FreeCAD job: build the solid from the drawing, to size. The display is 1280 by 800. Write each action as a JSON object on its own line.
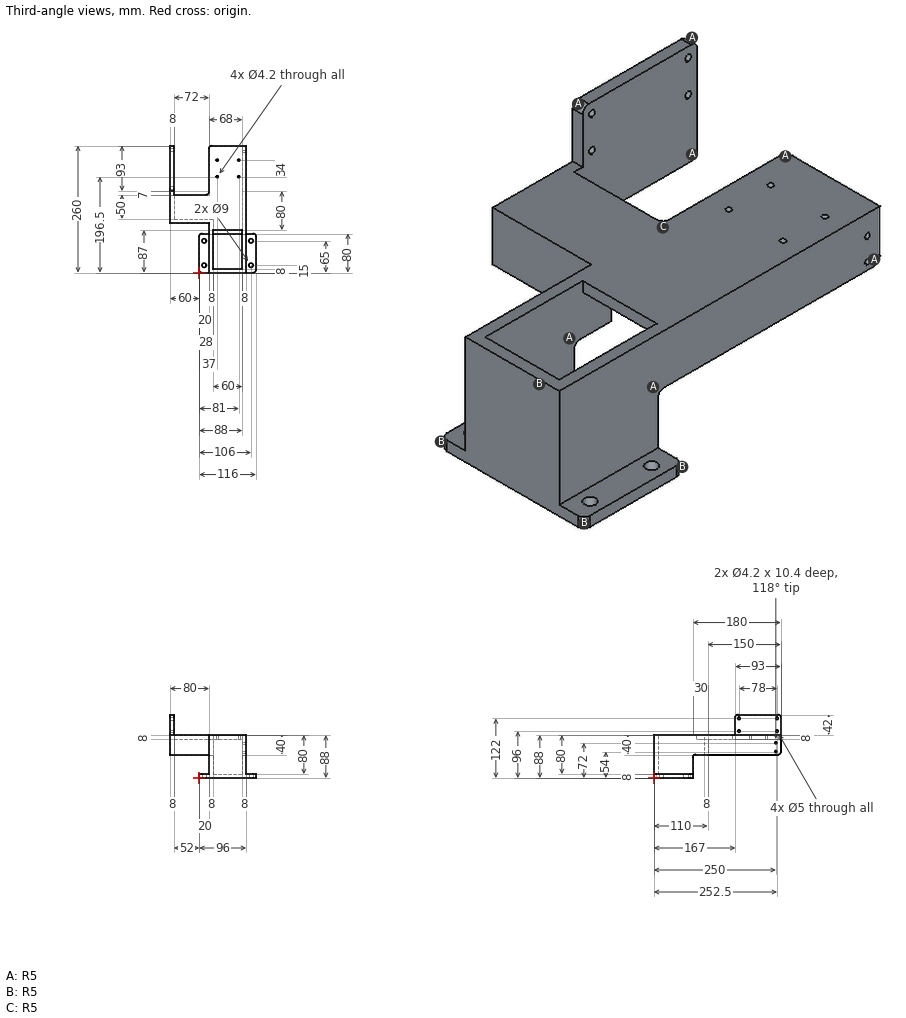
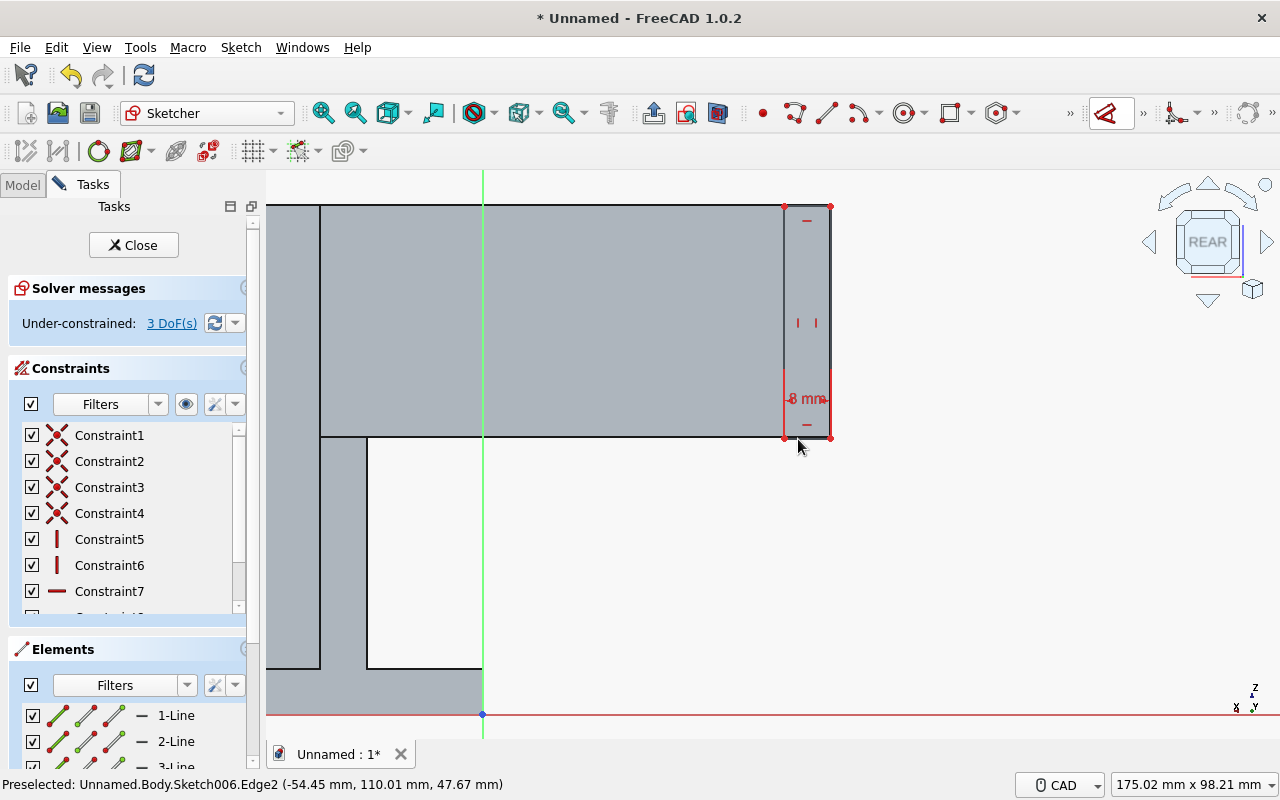
{"action": "left_click", "coordinate": [784, 276]}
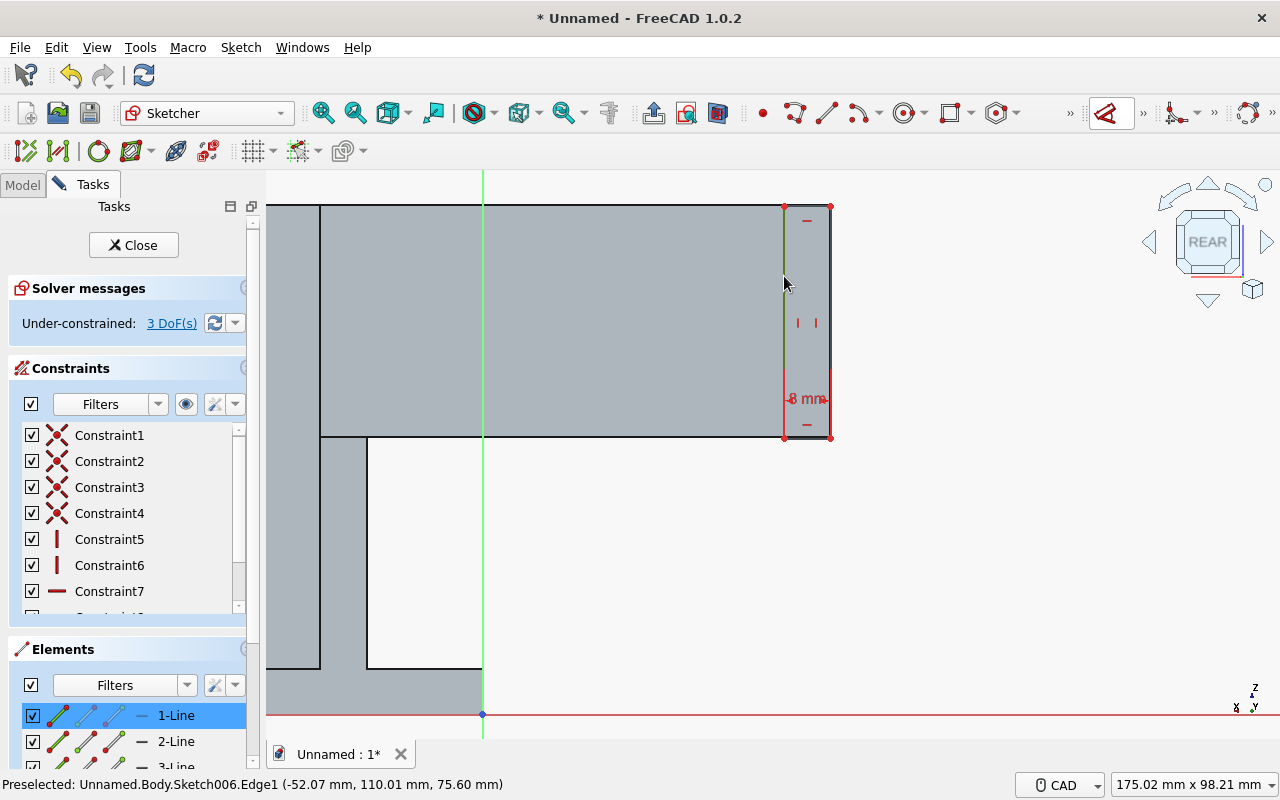
{"action": "key", "text": "i"}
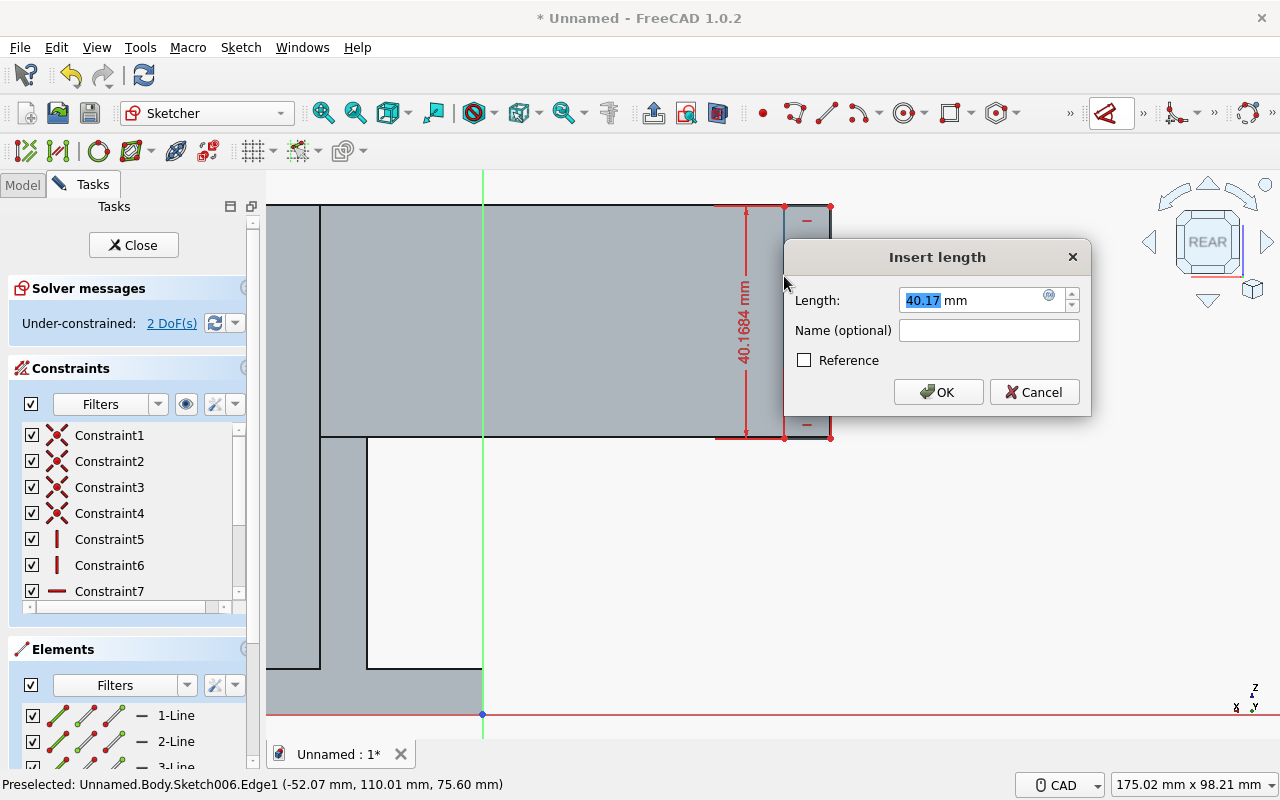
{"action": "type", "text": "40"}
{"action": "key", "text": "Return"}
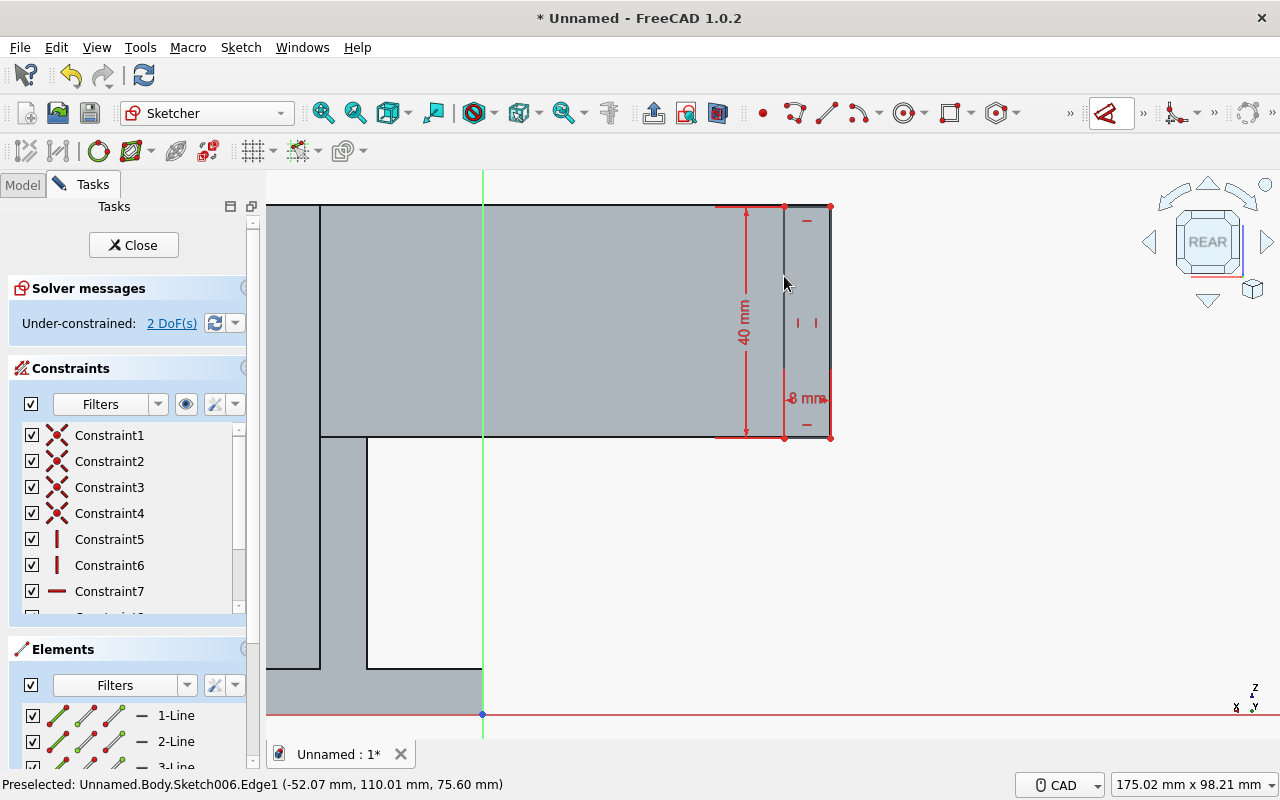
{"action": "left_click", "coordinate": [784, 207]}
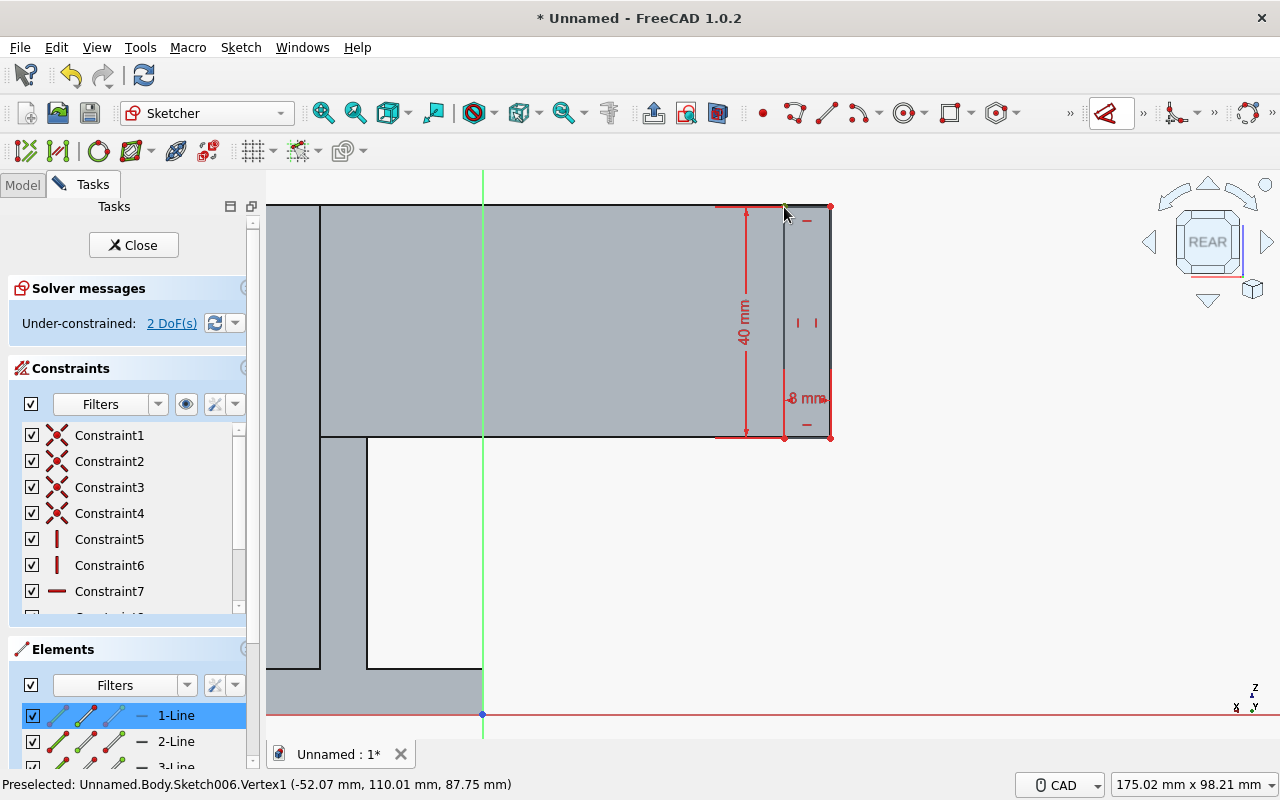
{"action": "key", "text": "l"}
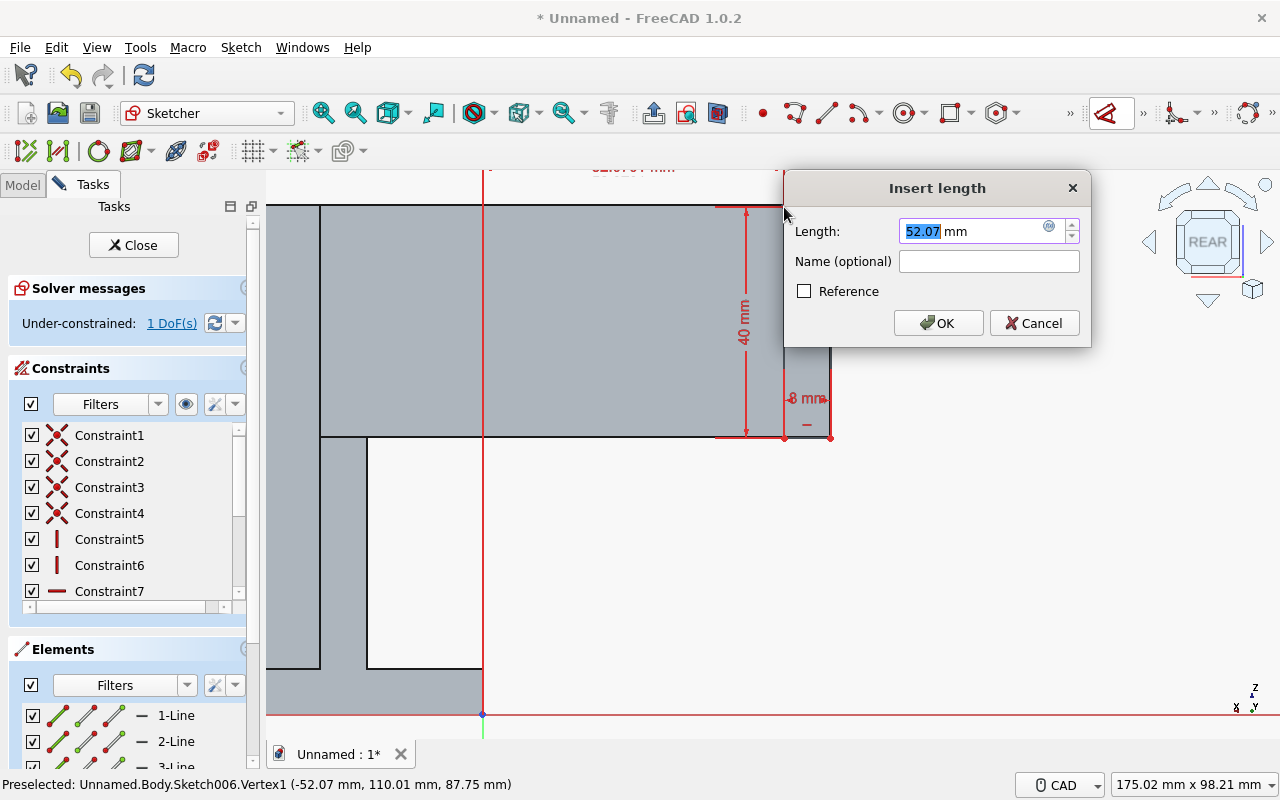
{"action": "type", "text": "52"}
{"action": "key", "text": "Return"}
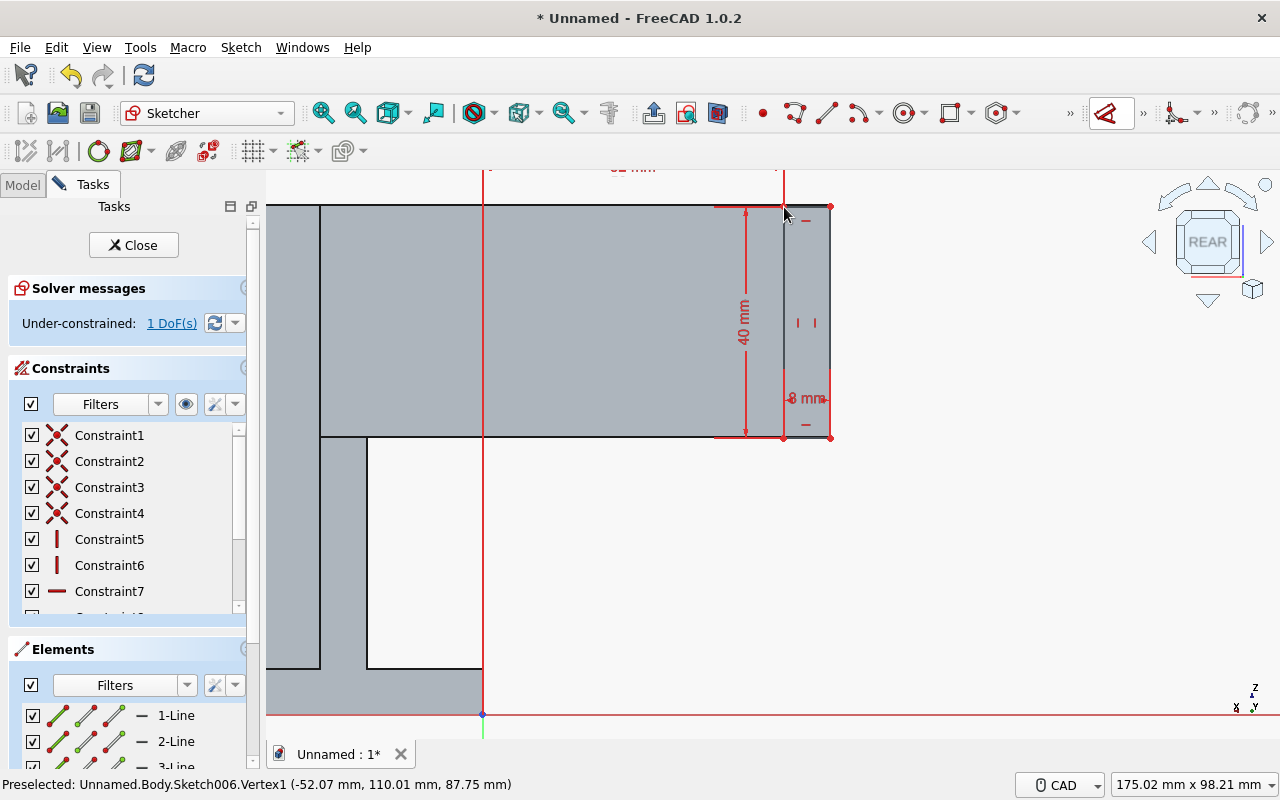
{"action": "left_click", "coordinate": [784, 207]}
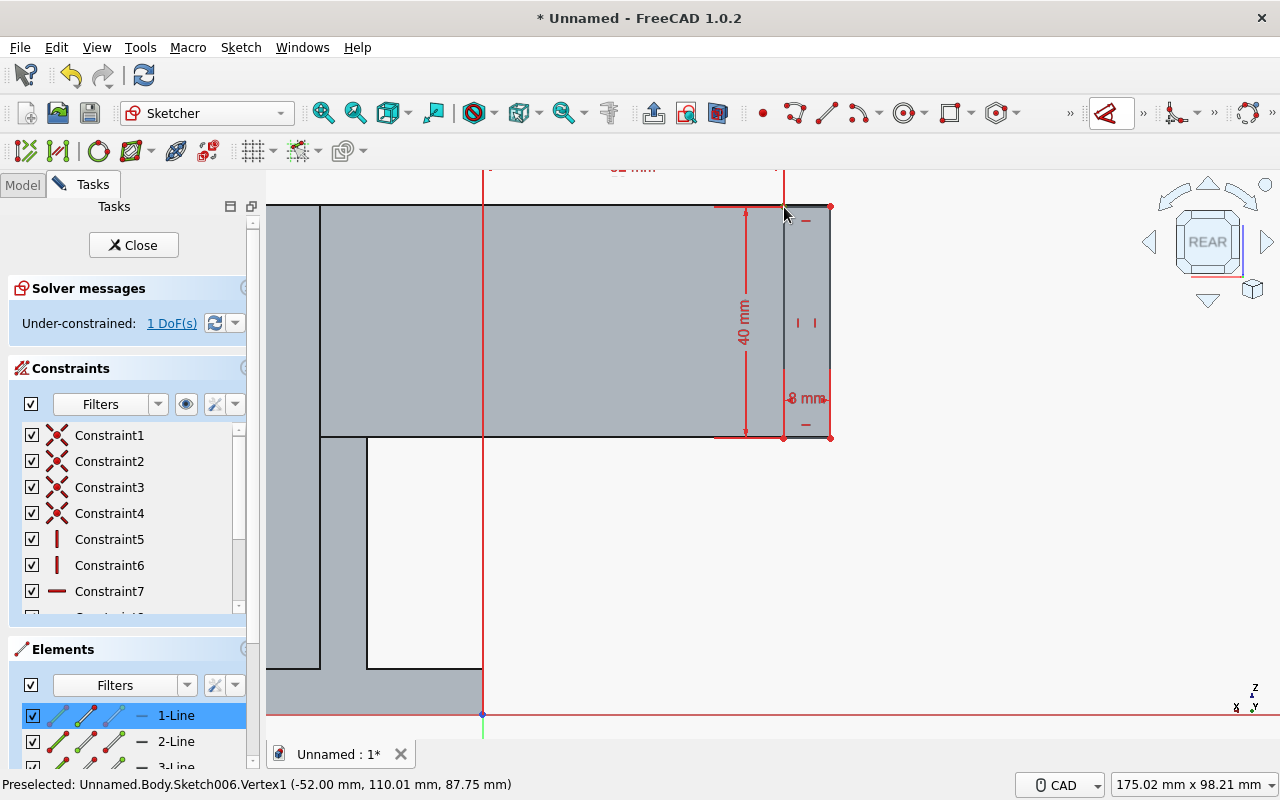
{"action": "left_click", "coordinate": [1128, 114]}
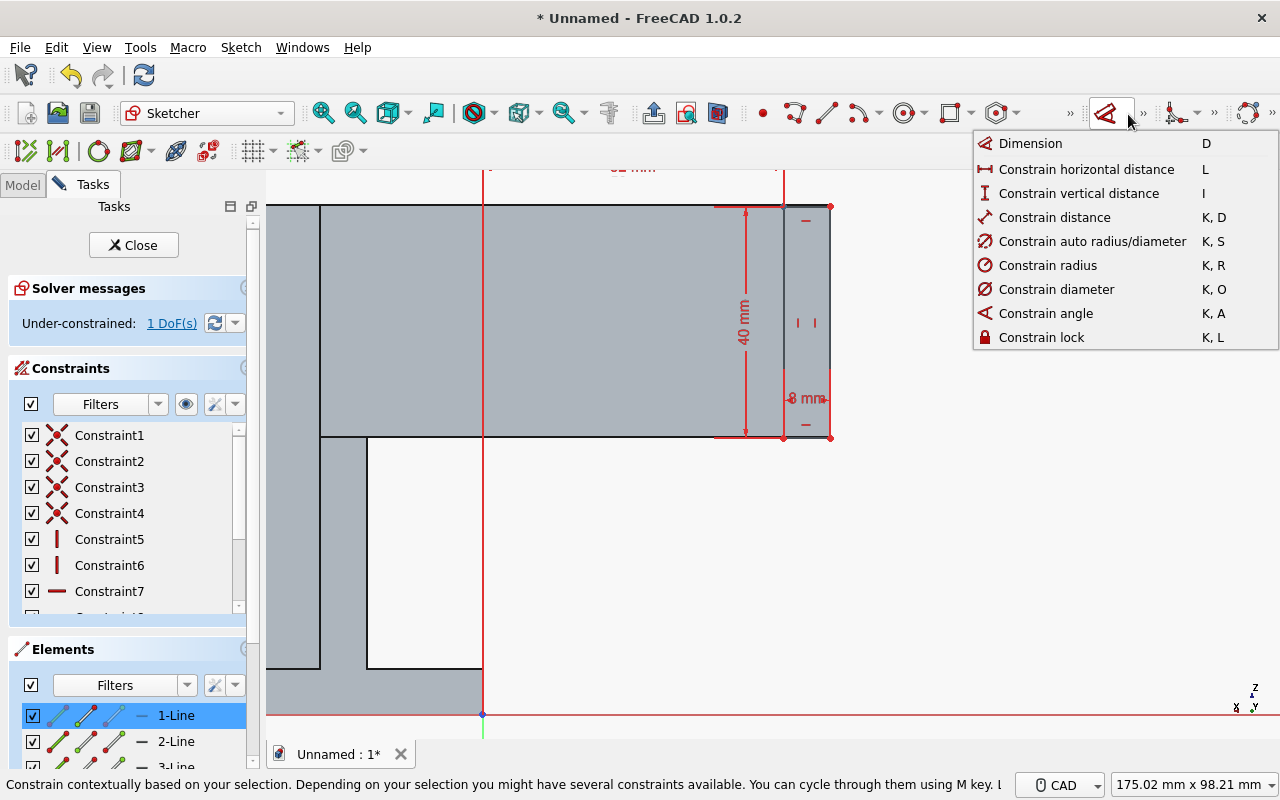
{"action": "left_click", "coordinate": [1126, 193]}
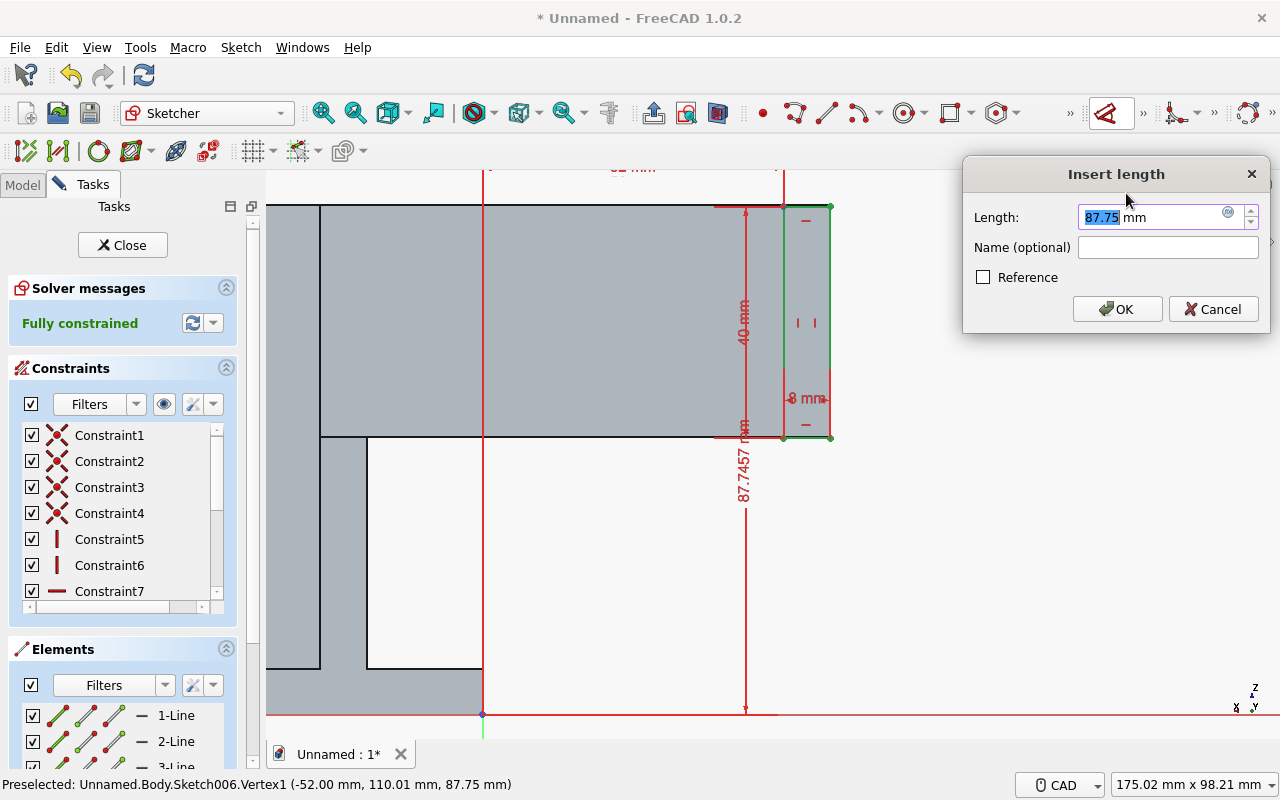
{"action": "type", "text": "88"}
{"action": "key", "text": "Return"}